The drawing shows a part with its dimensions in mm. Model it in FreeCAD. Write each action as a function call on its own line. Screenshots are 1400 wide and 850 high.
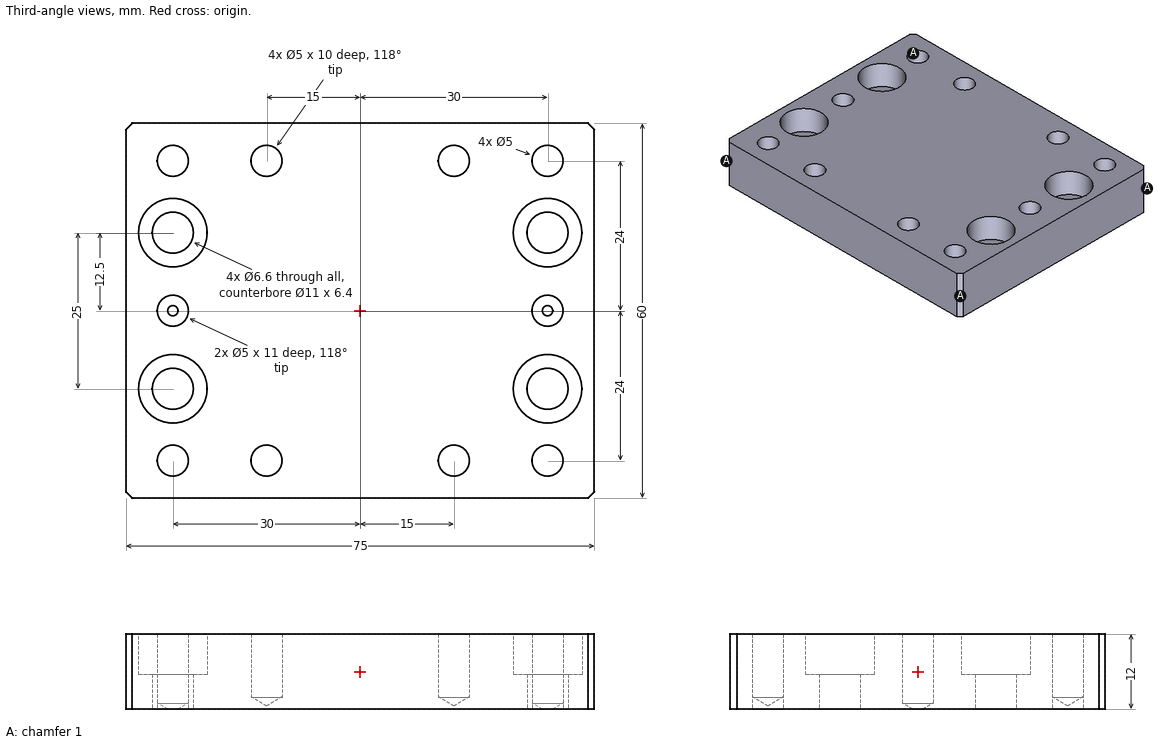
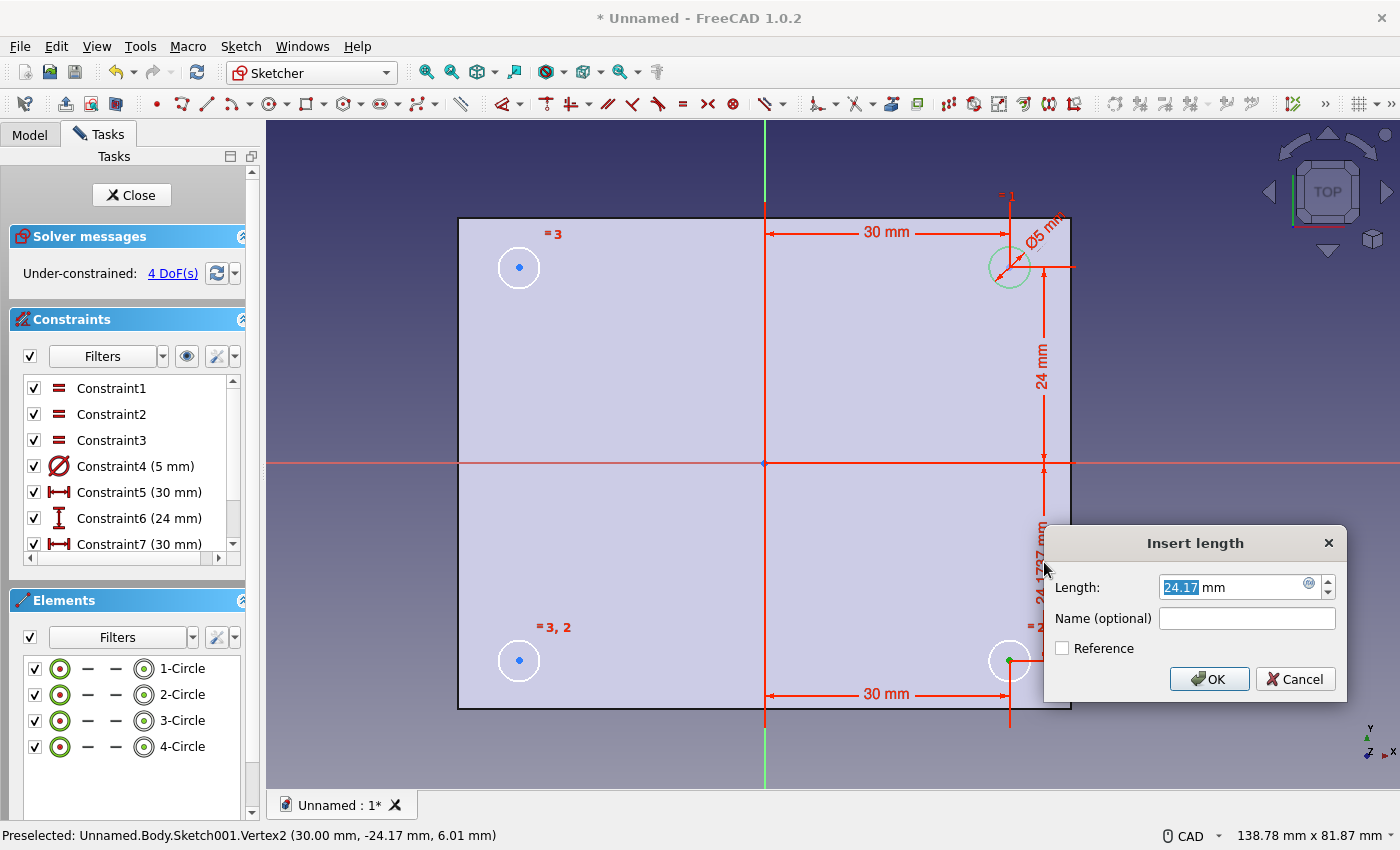
text(24)
key(Return)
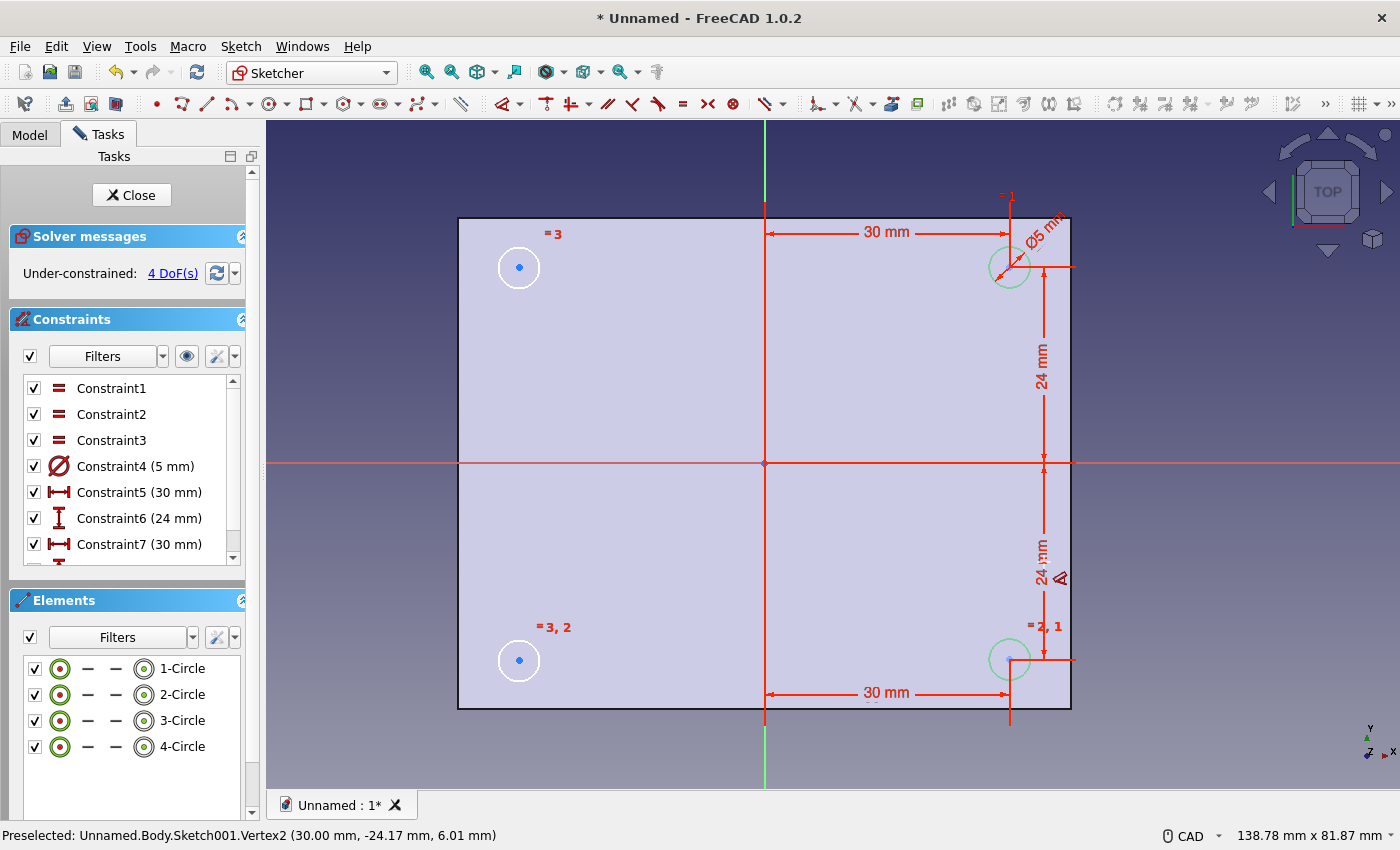
click(519, 661)
click(642, 695)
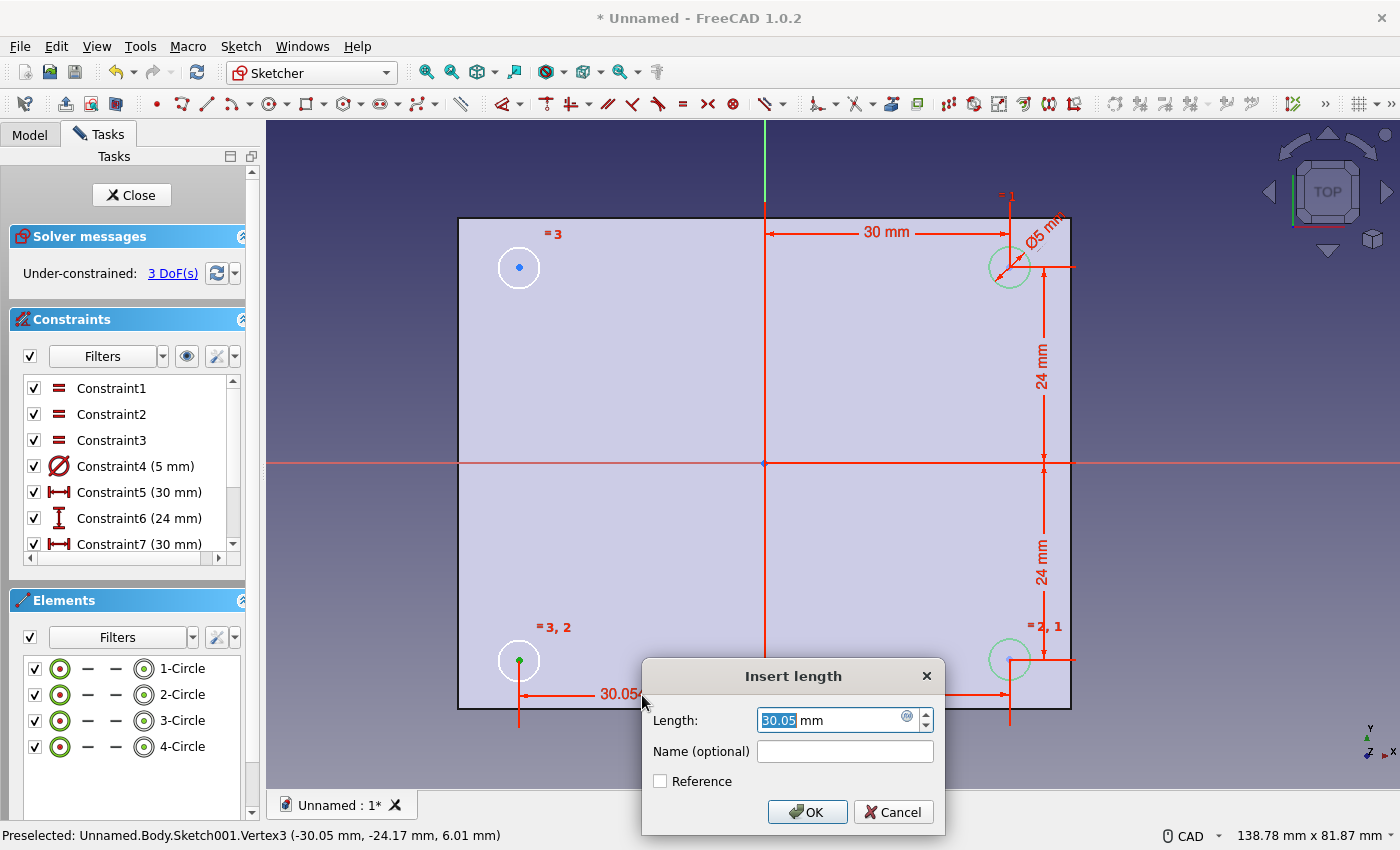
text(30)
key(Return)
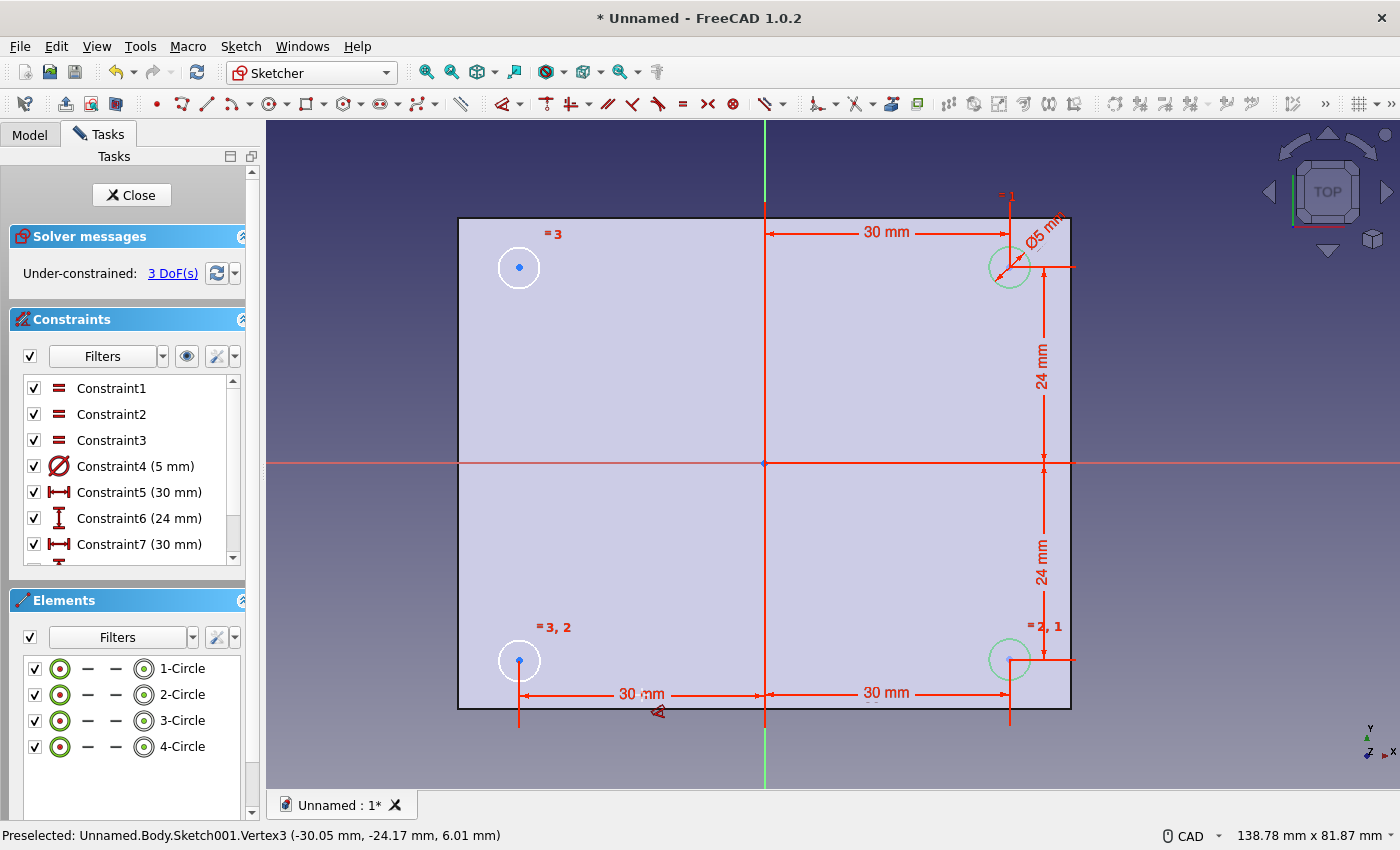
click(519, 661)
click(485, 562)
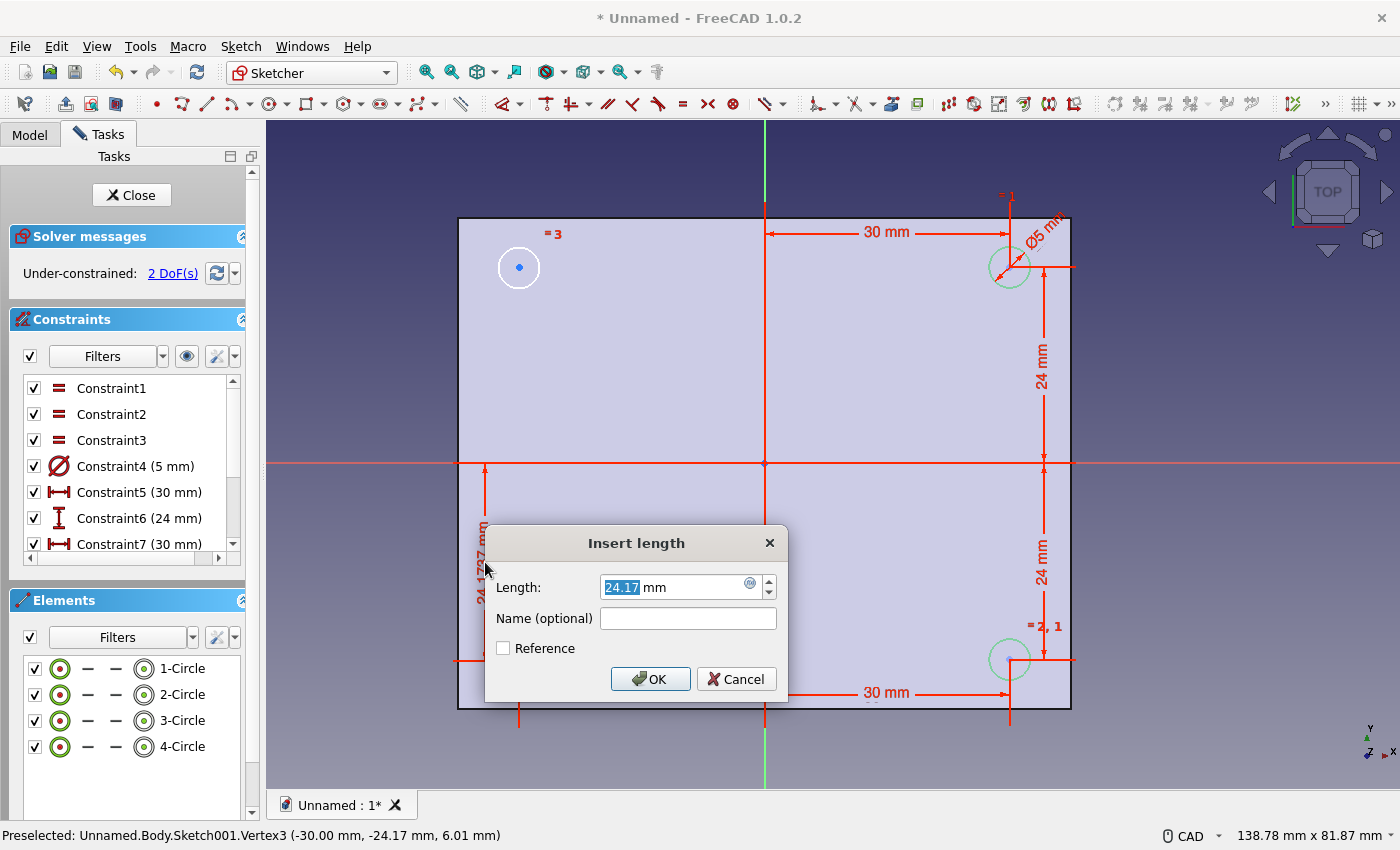
text(24)
key(Return)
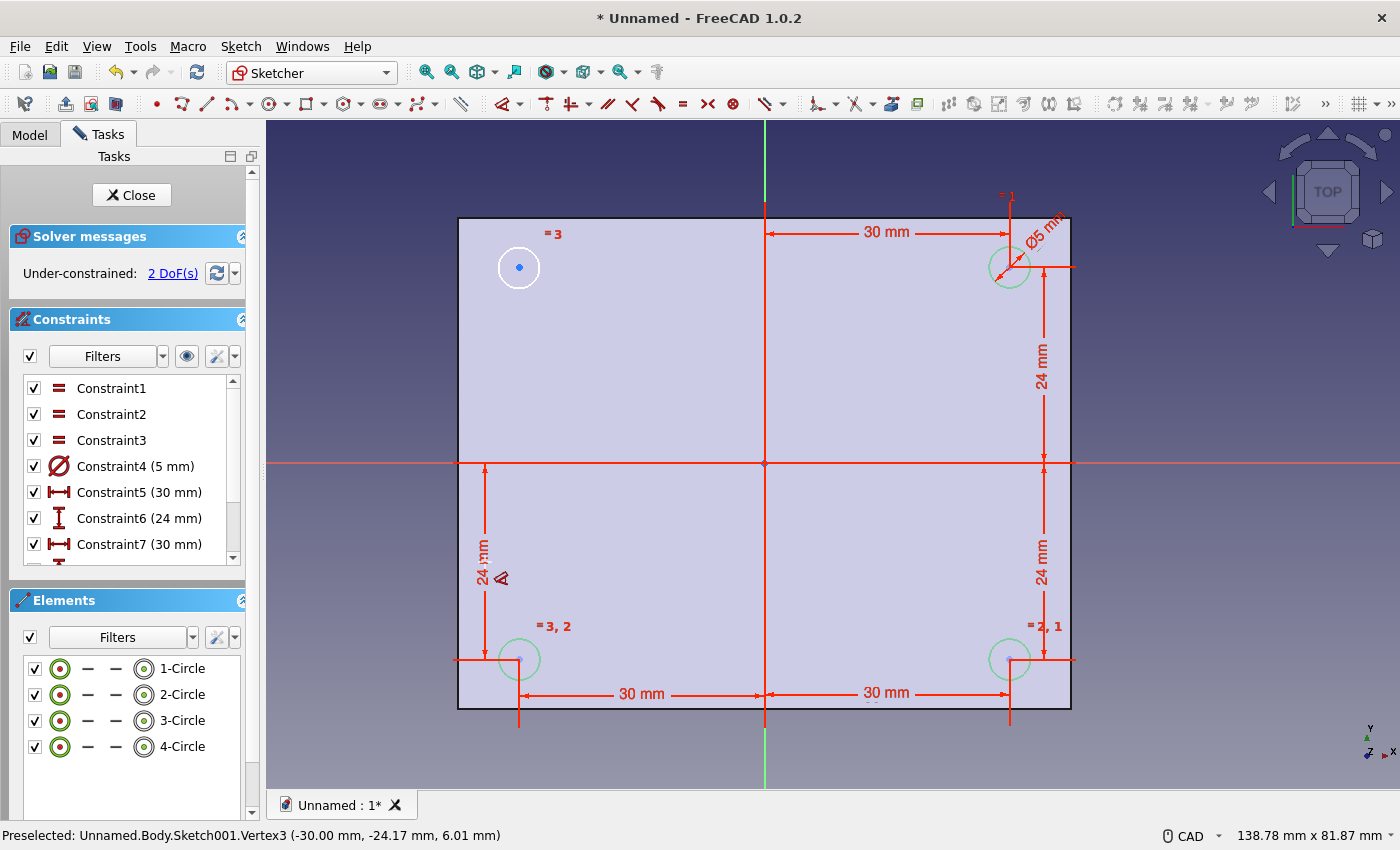
click(519, 268)
click(642, 234)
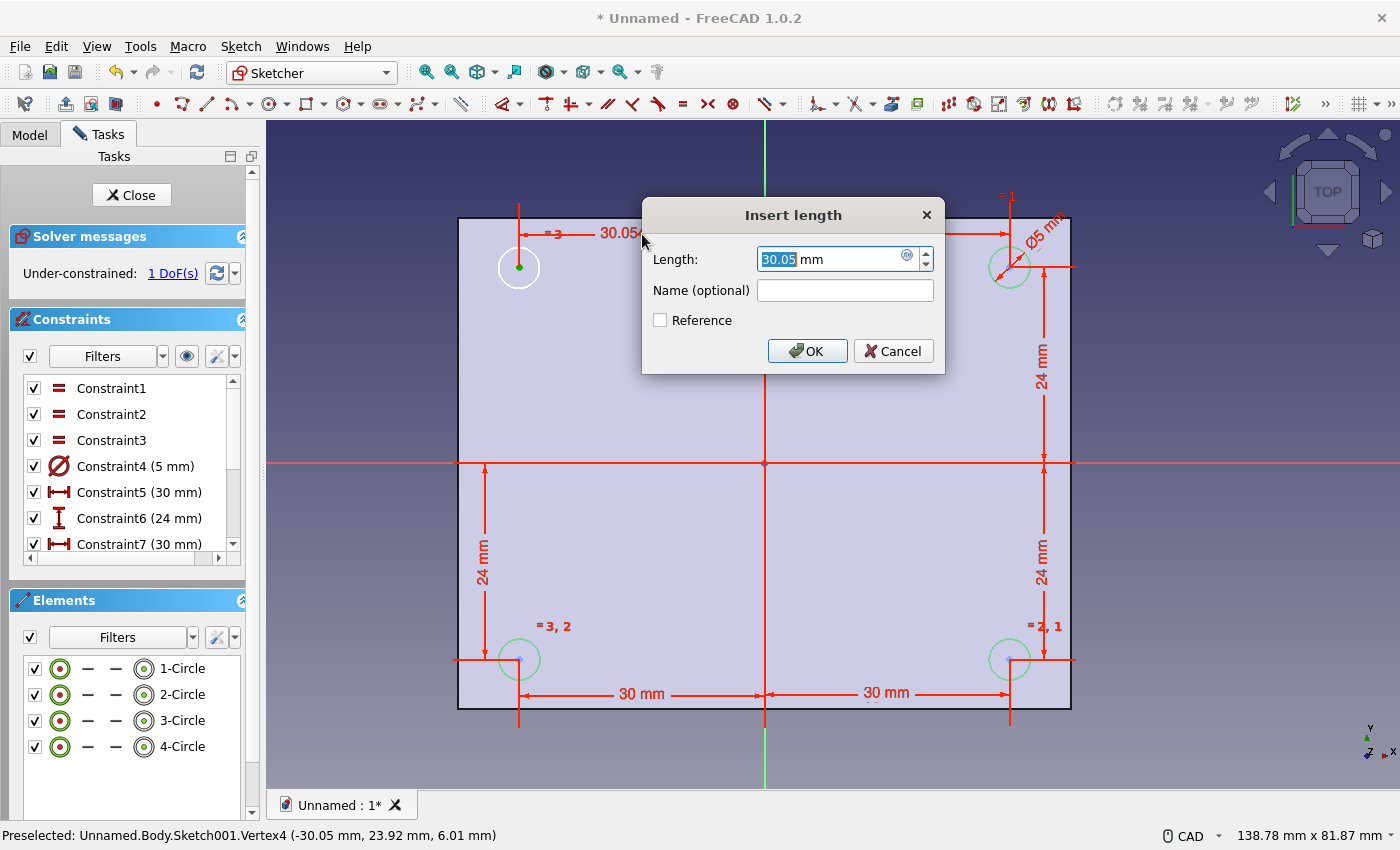
text(30)
key(Return)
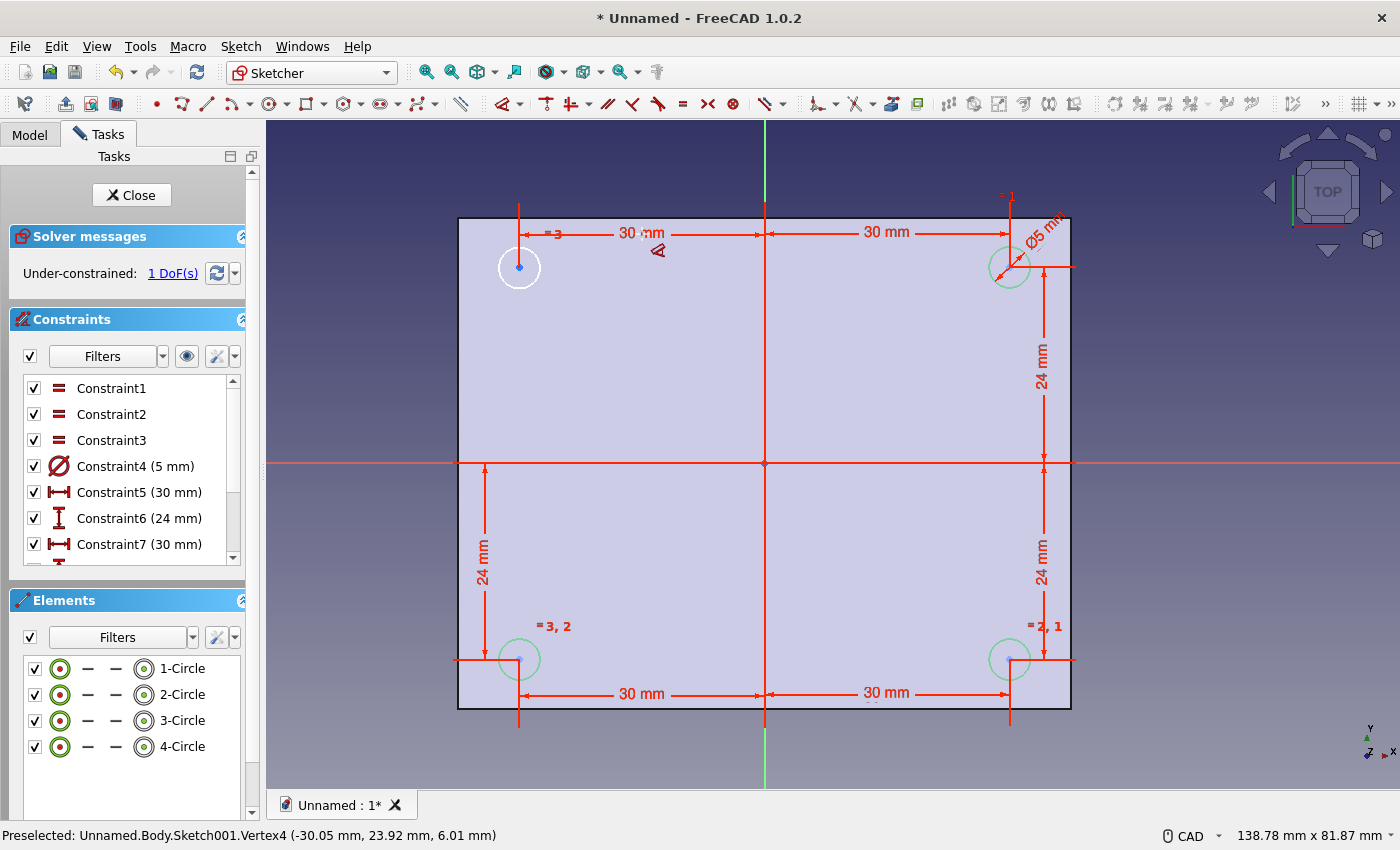
click(519, 268)
click(485, 366)